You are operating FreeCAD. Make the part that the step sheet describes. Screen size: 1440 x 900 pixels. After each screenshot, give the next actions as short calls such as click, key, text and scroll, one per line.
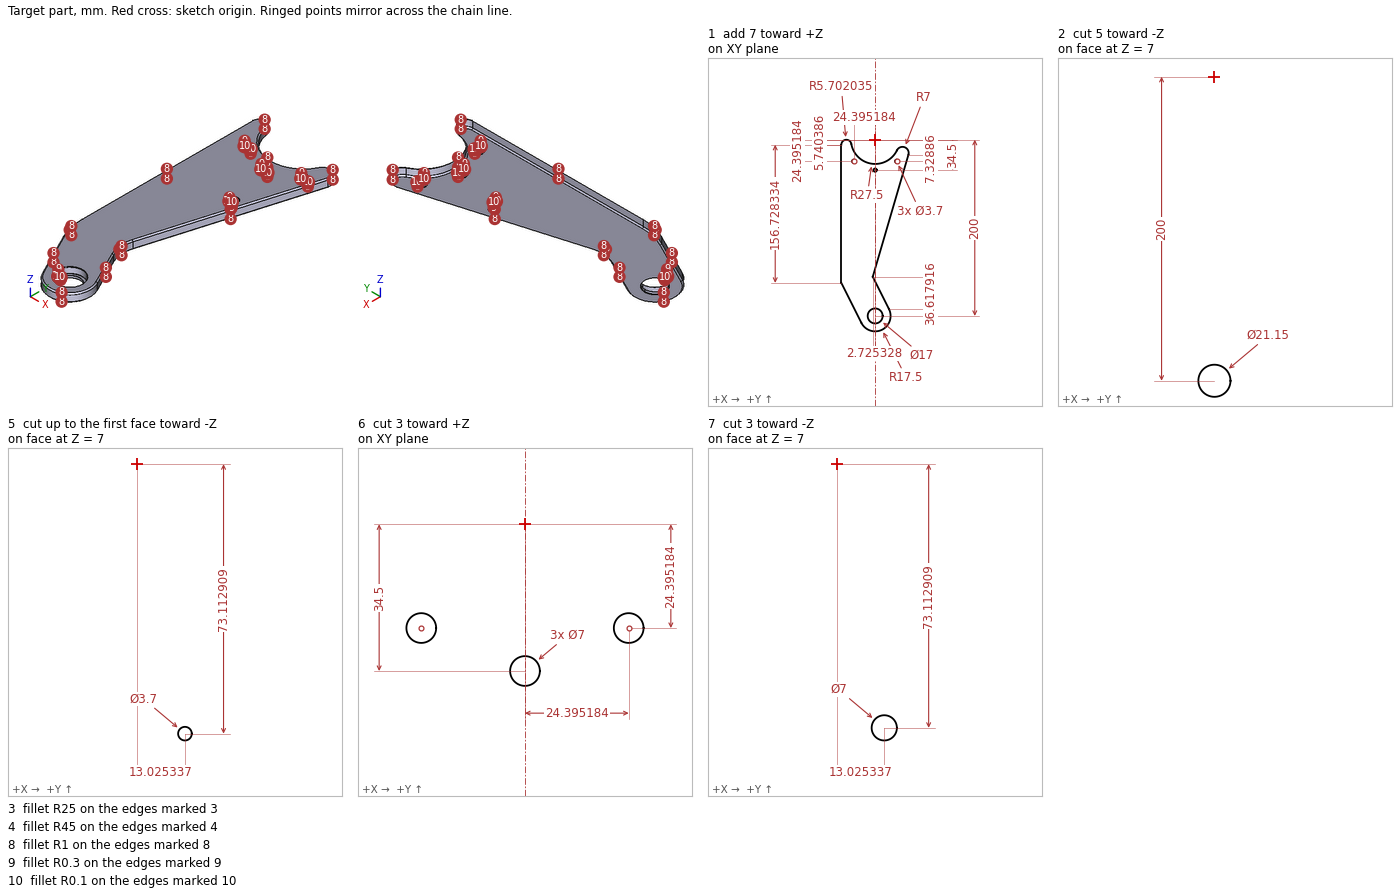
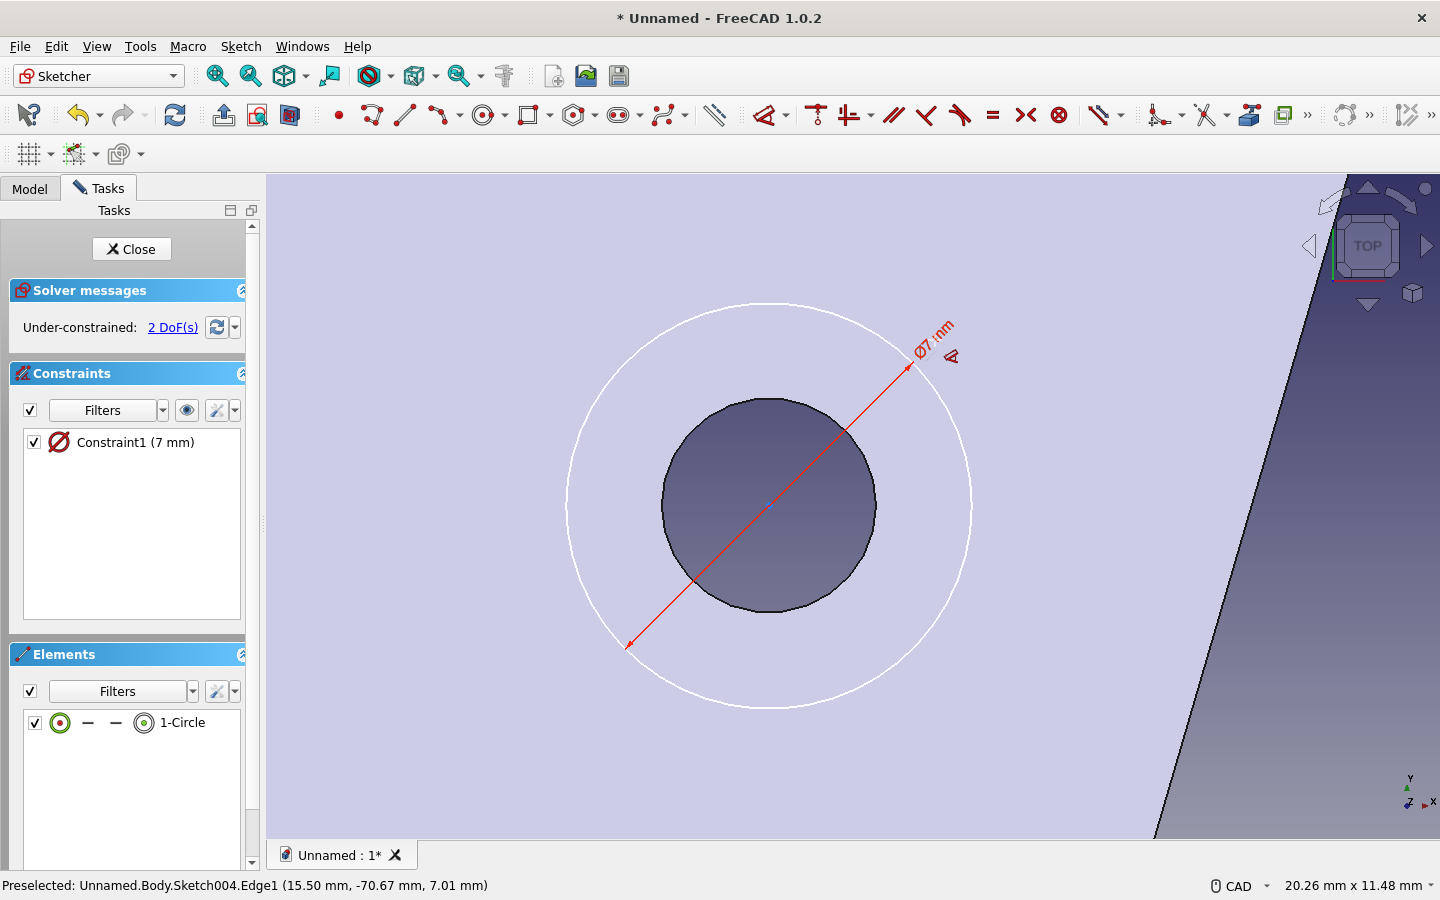
click(769, 506)
click(532, 540)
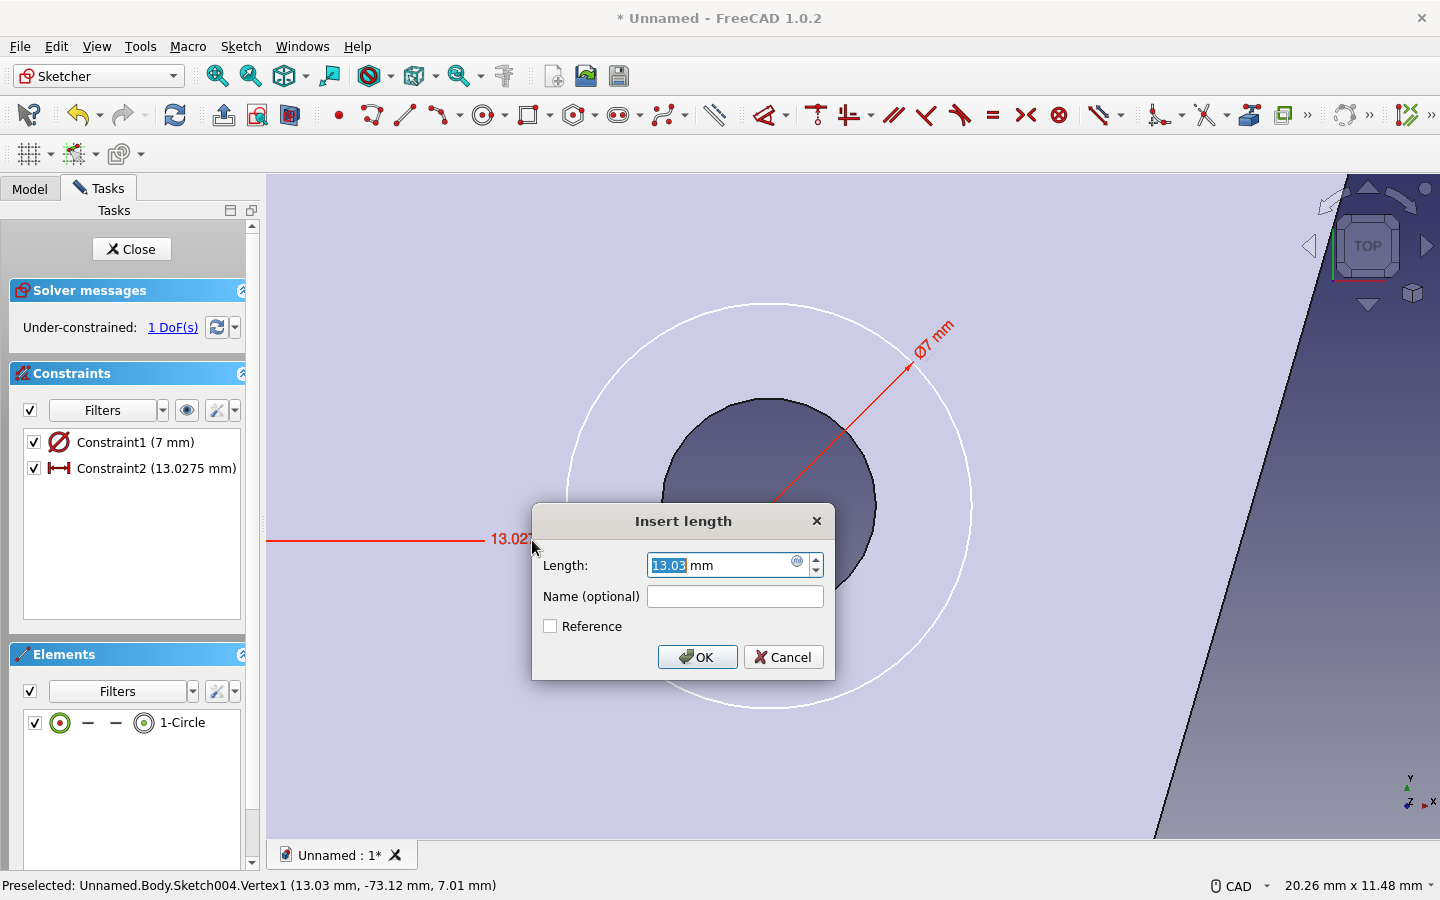
text(13.025337)
key(Return)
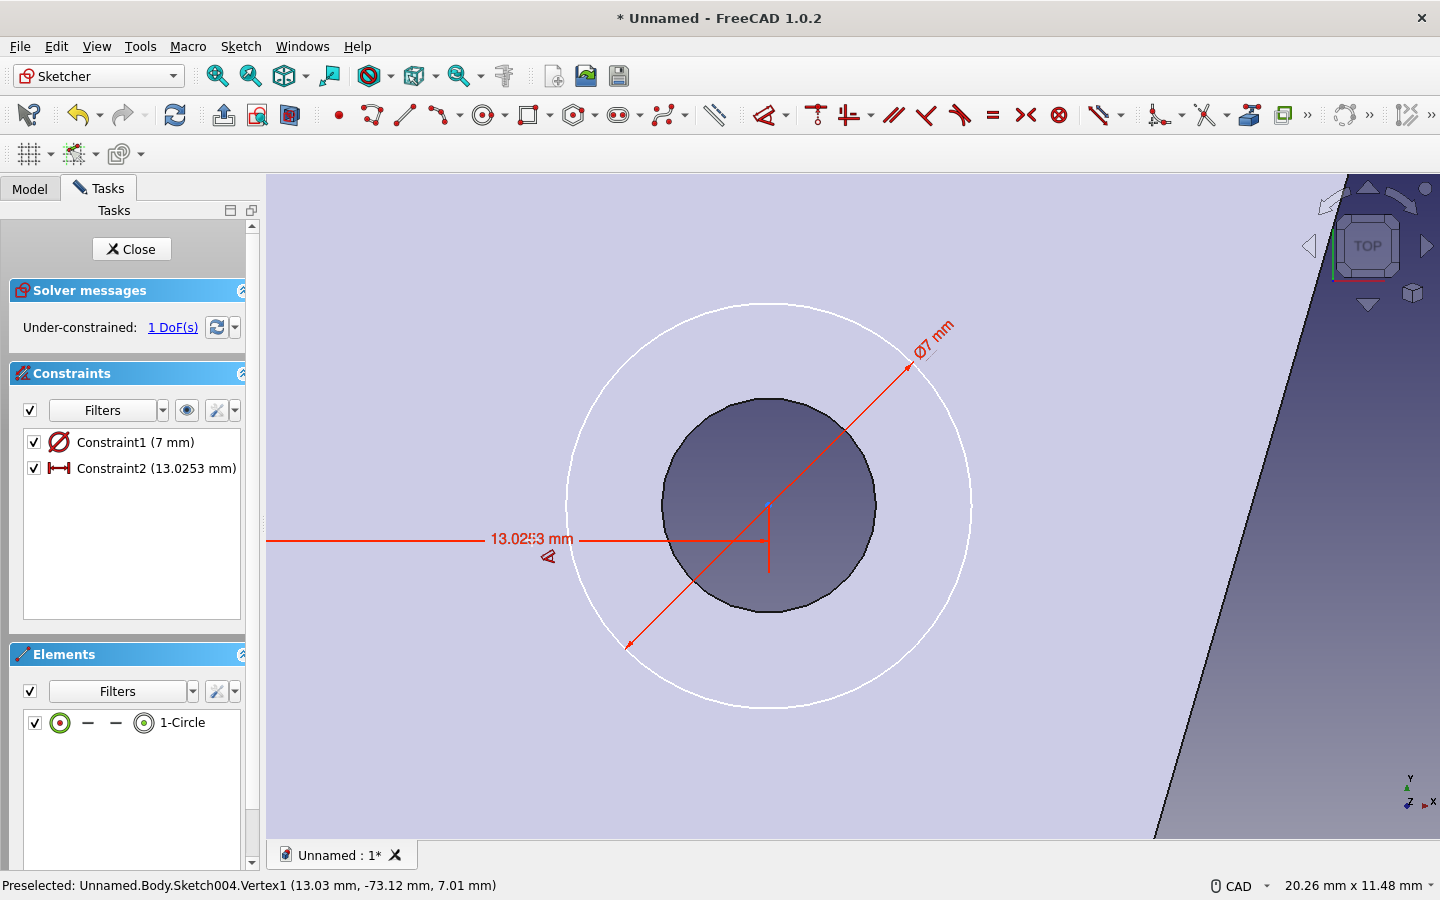
click(769, 506)
click(803, 354)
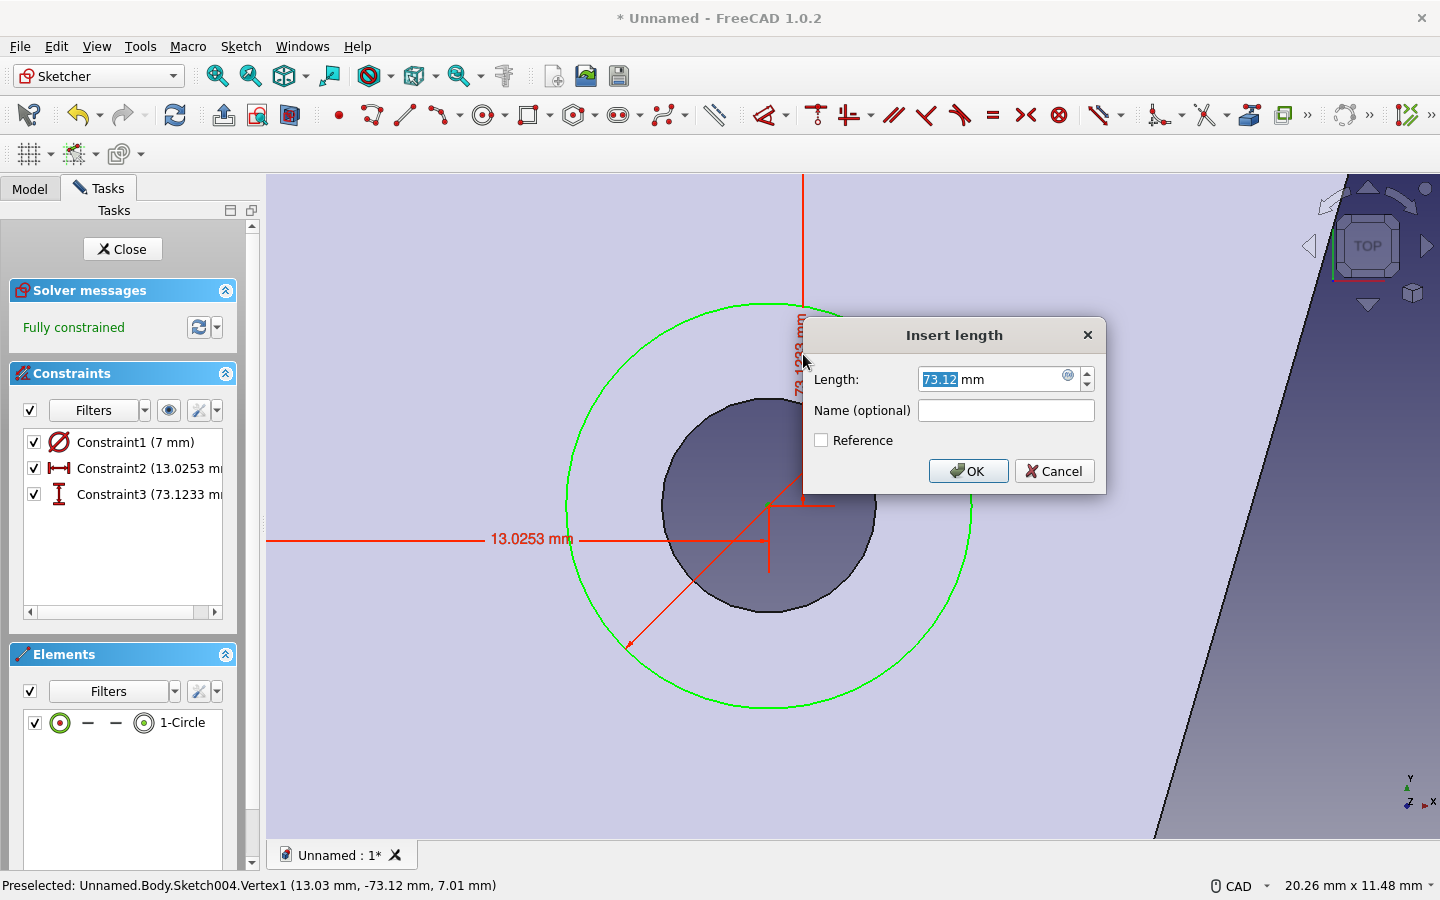
text(73.112909)
key(Return)
key(Escape)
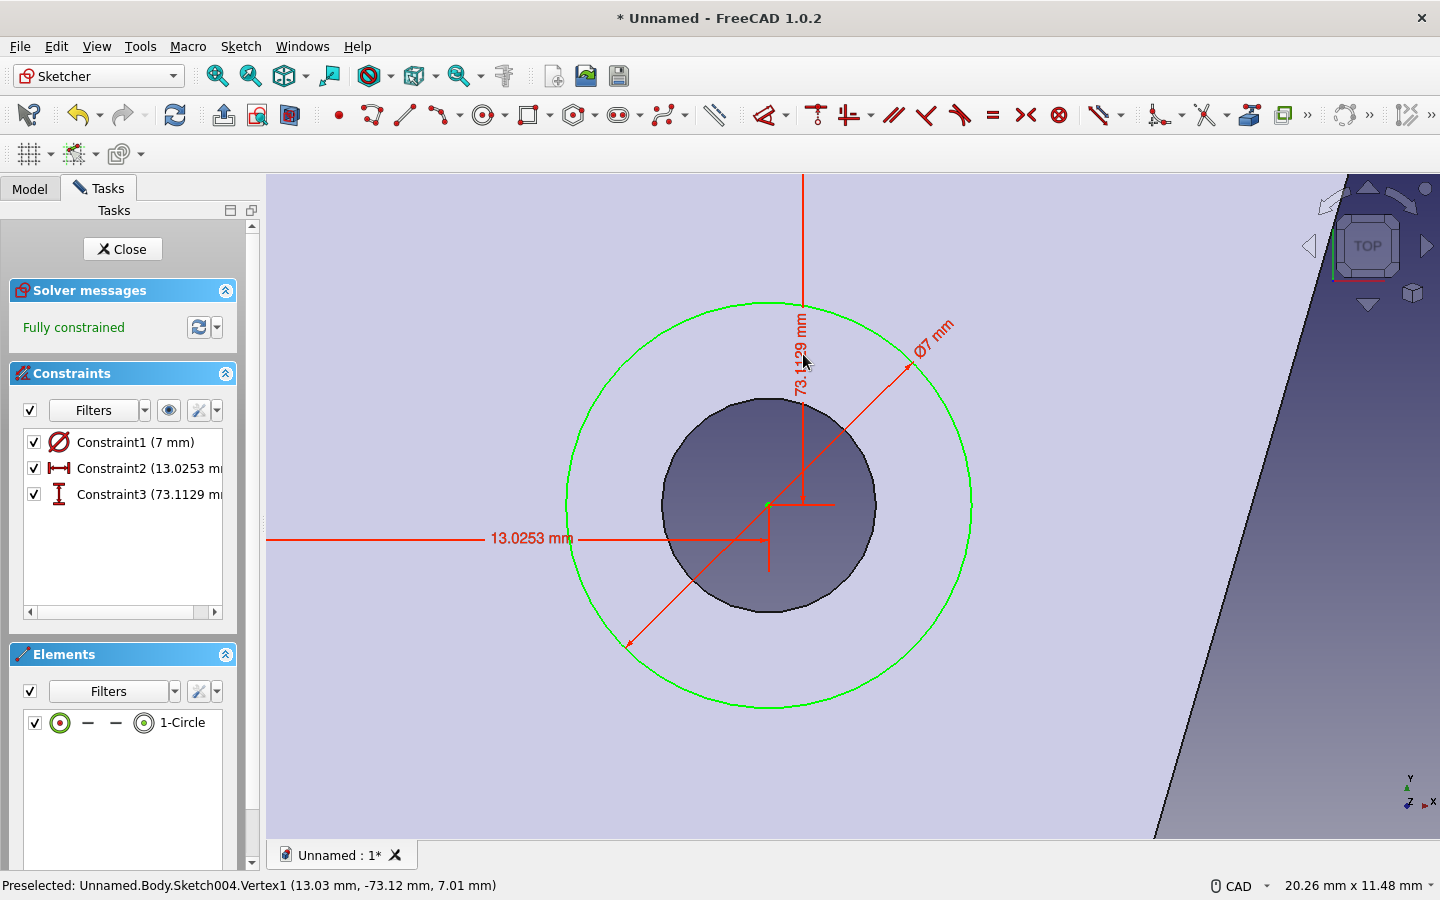
click(123, 249)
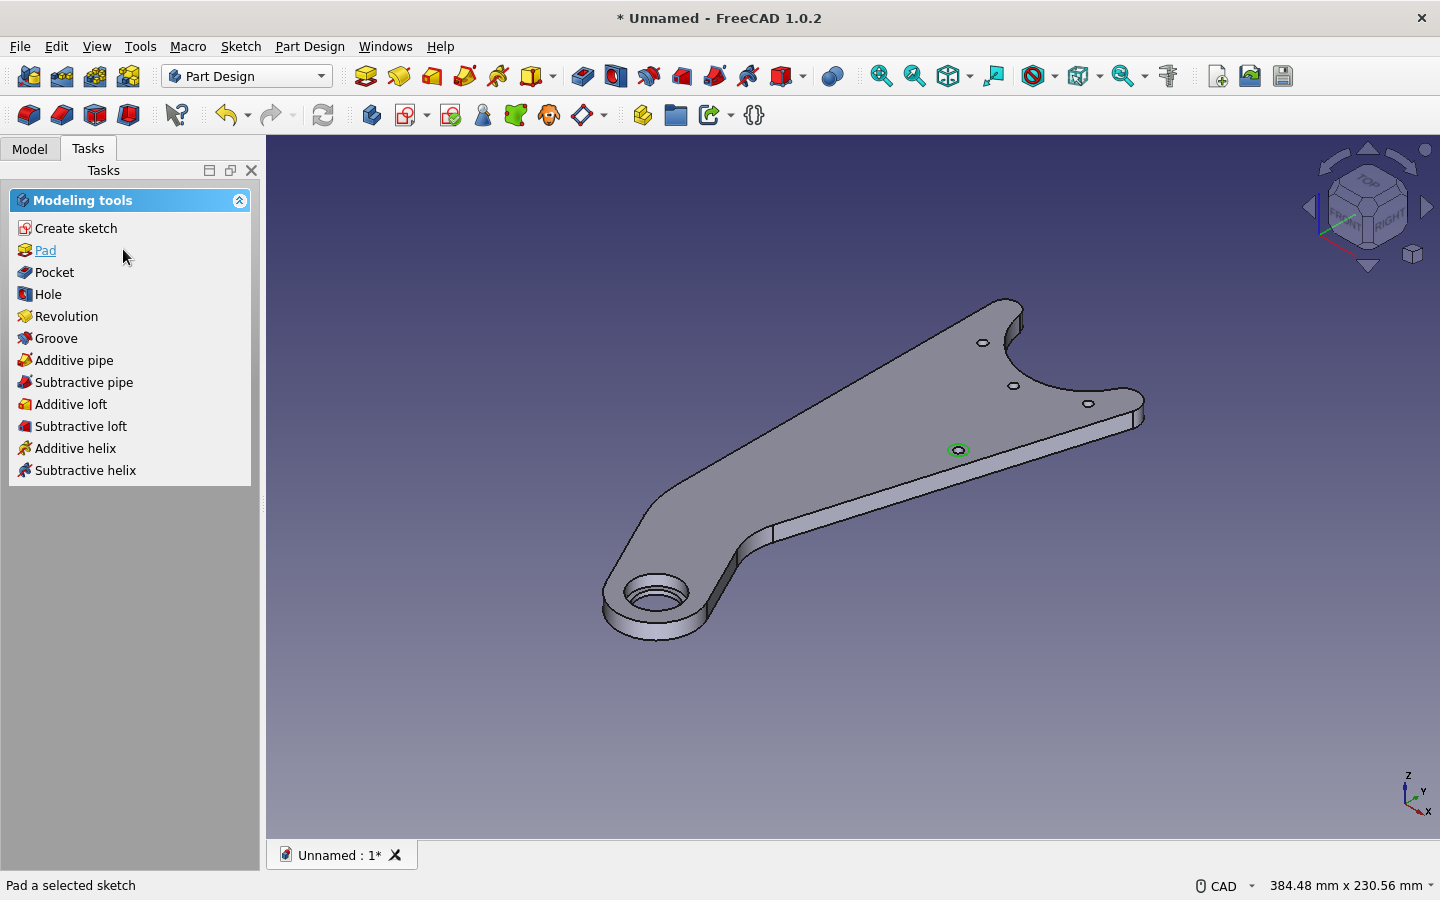
click(583, 76)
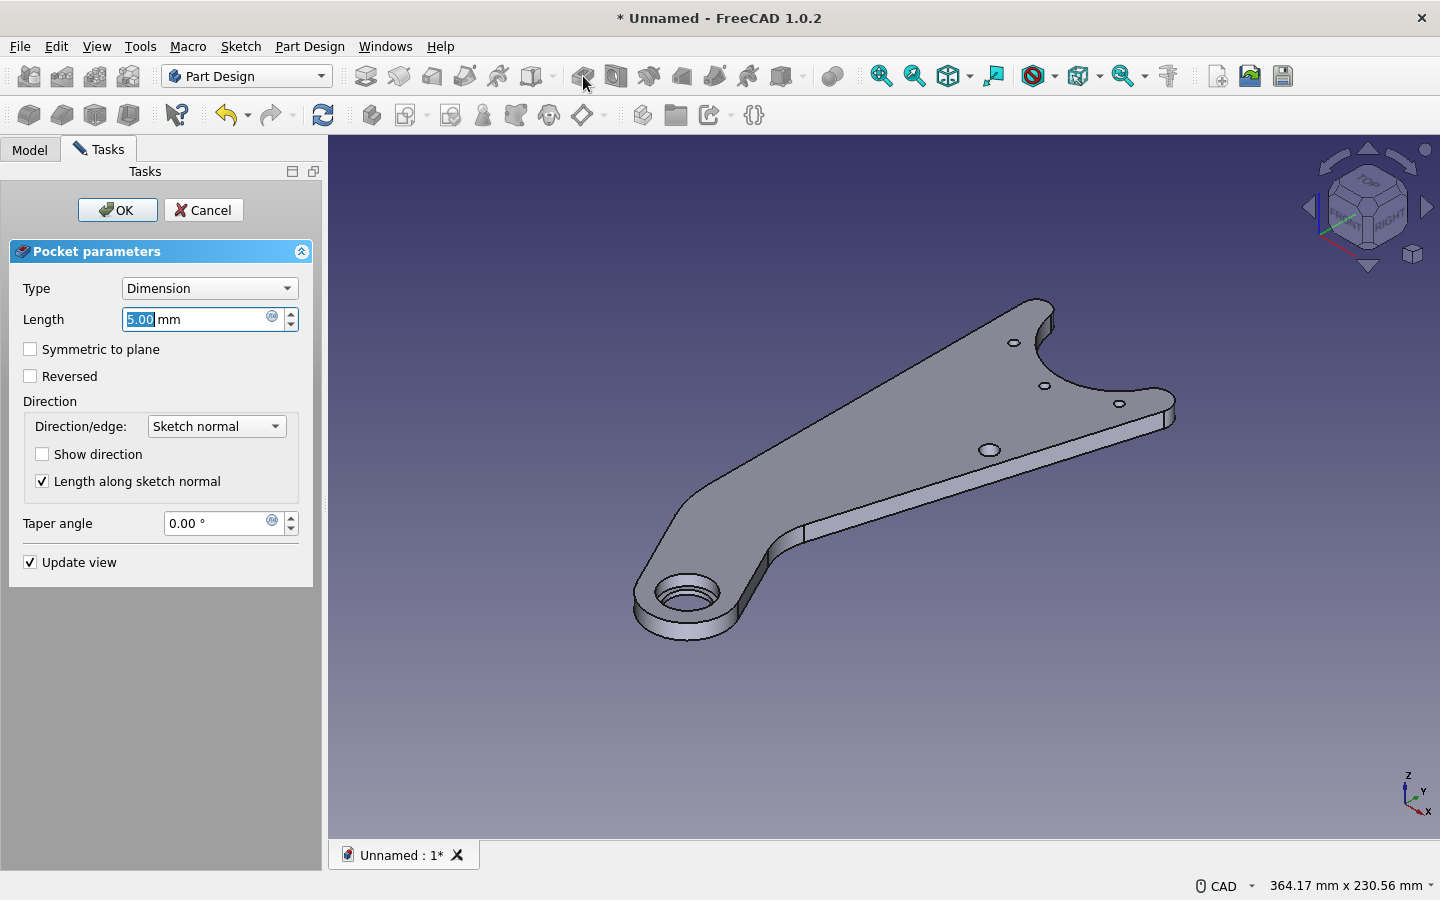
text(3)
key(Tab)